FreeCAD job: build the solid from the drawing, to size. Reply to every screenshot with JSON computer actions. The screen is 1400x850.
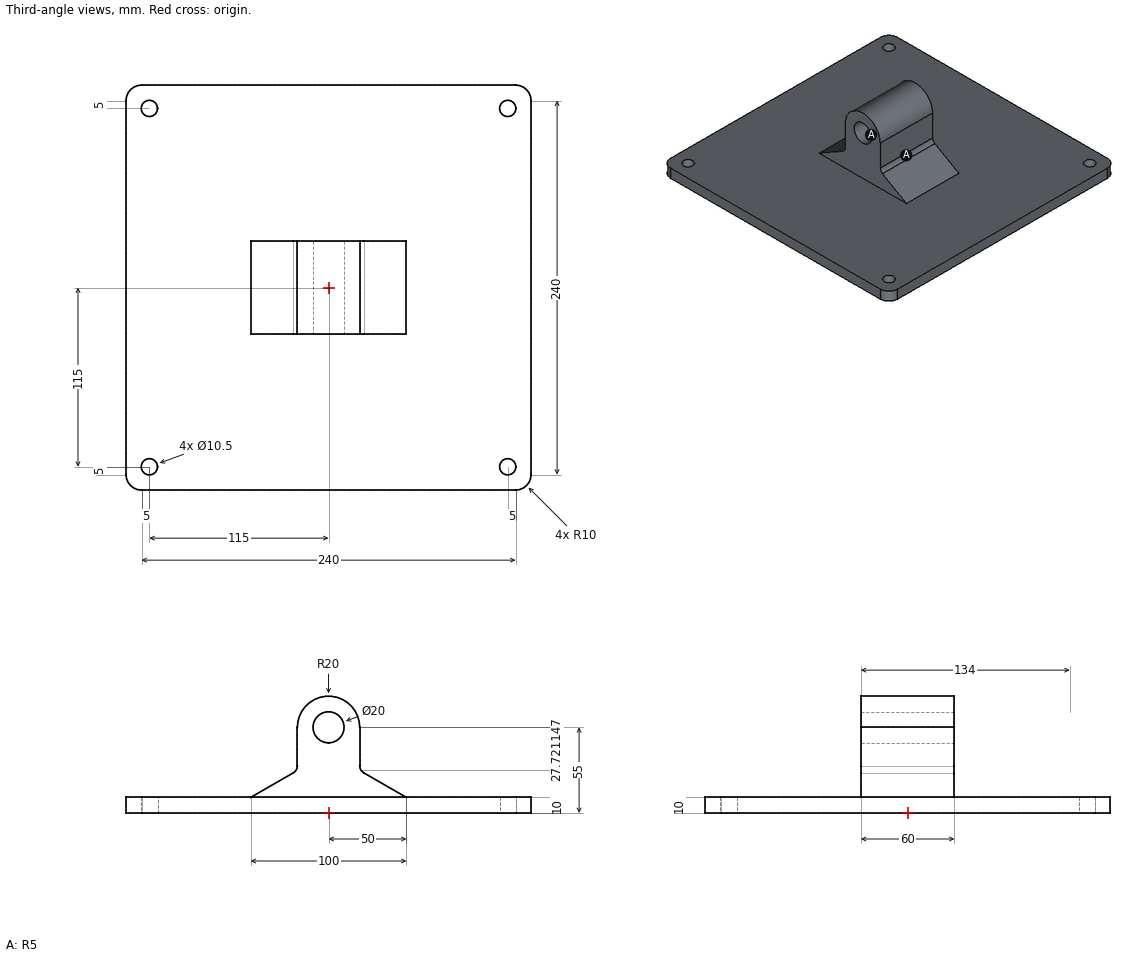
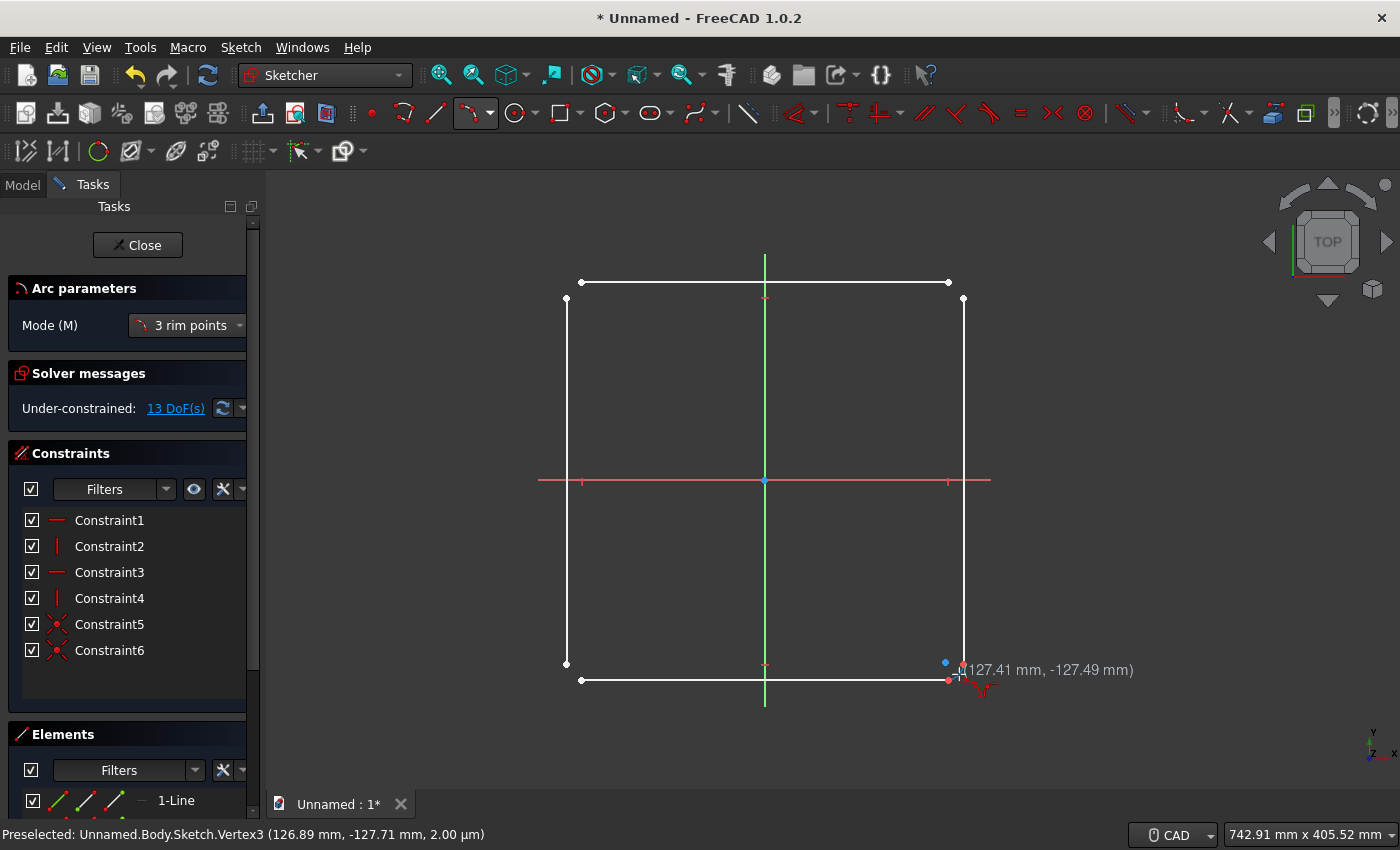
{"action": "left_click", "coordinate": [964, 298]}
{"action": "left_click", "coordinate": [949, 282]}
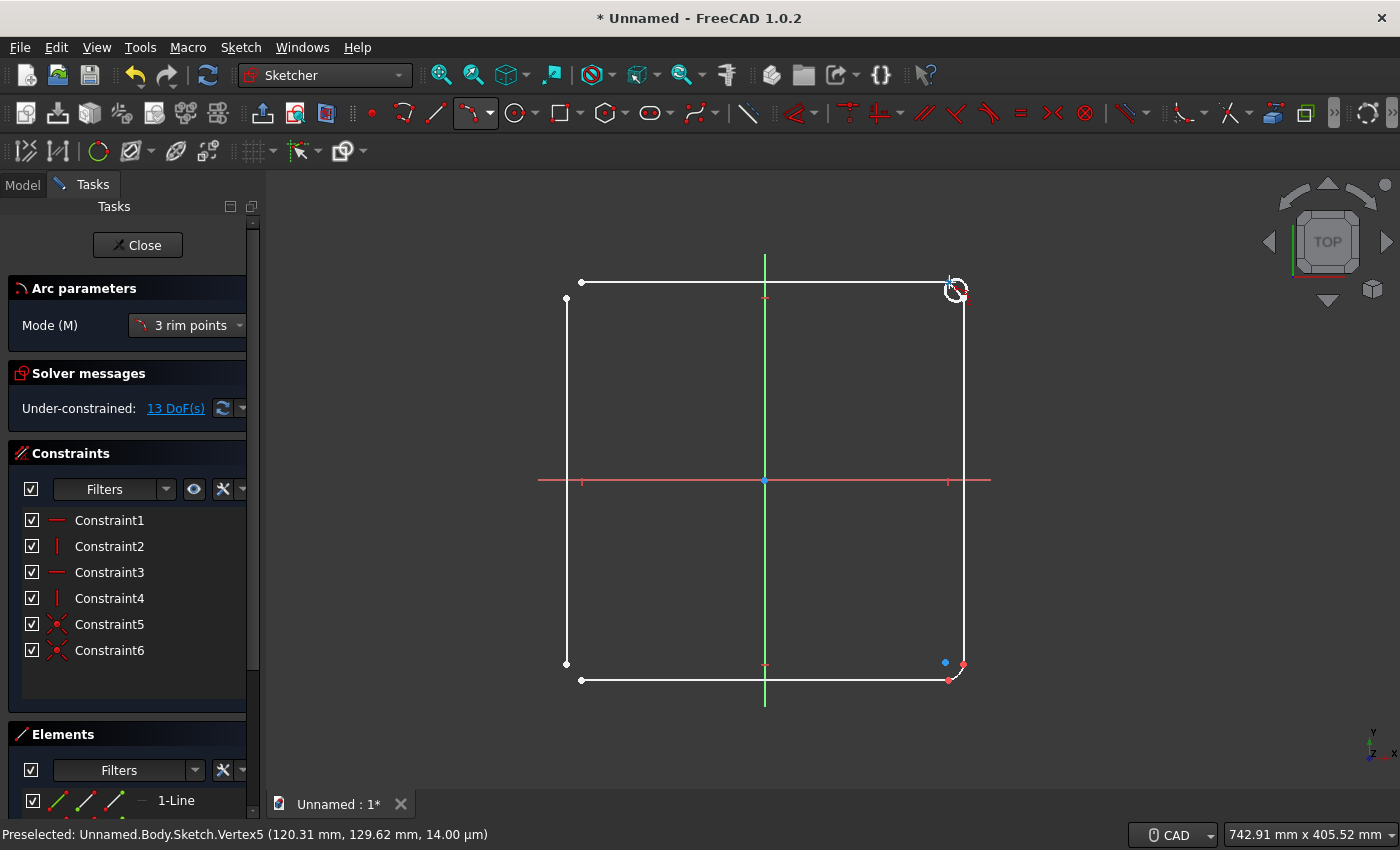
{"action": "scroll", "coordinate": [959, 286], "scroll_direction": "up", "scroll_amount": 7}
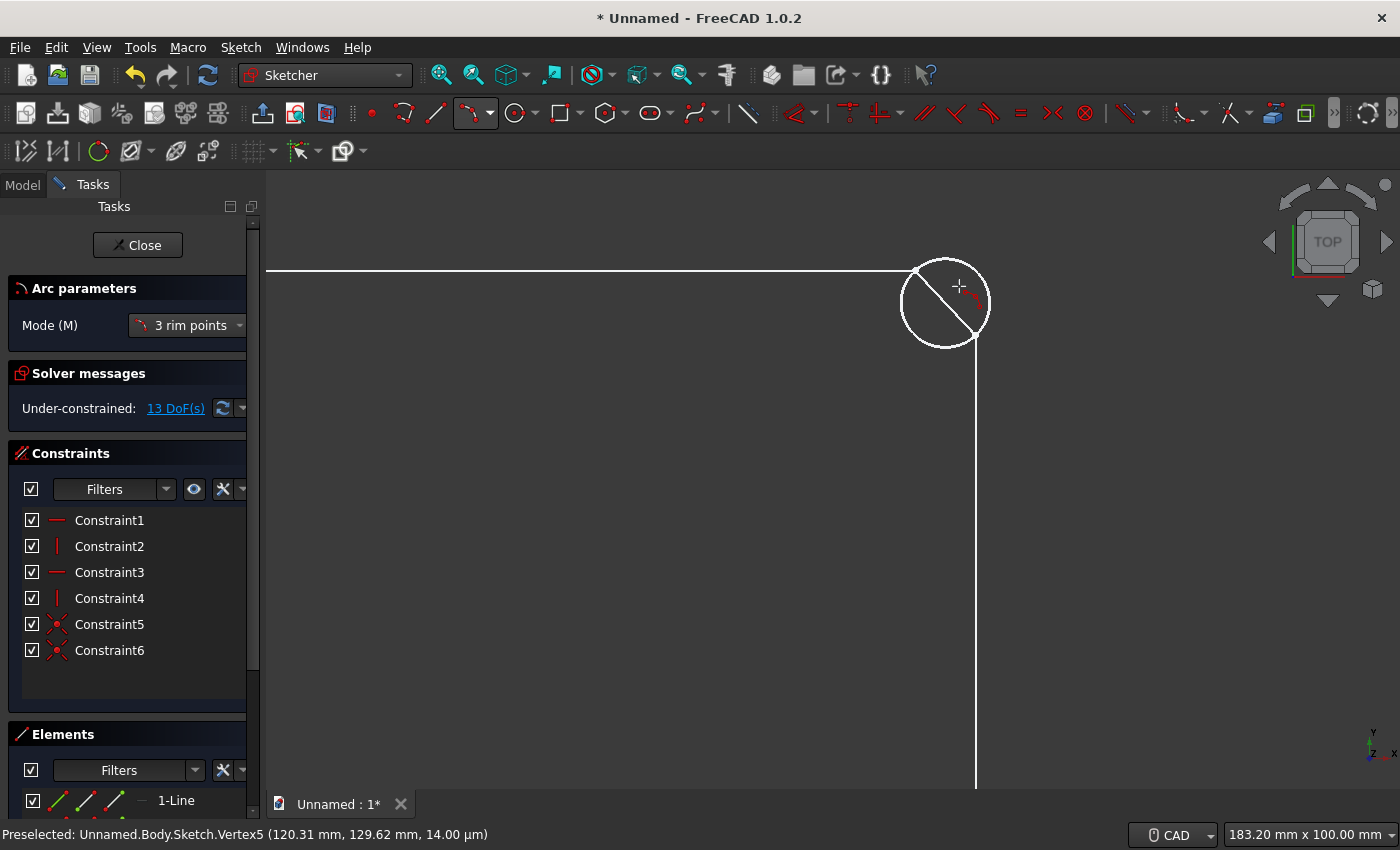
{"action": "left_click", "coordinate": [957, 287]}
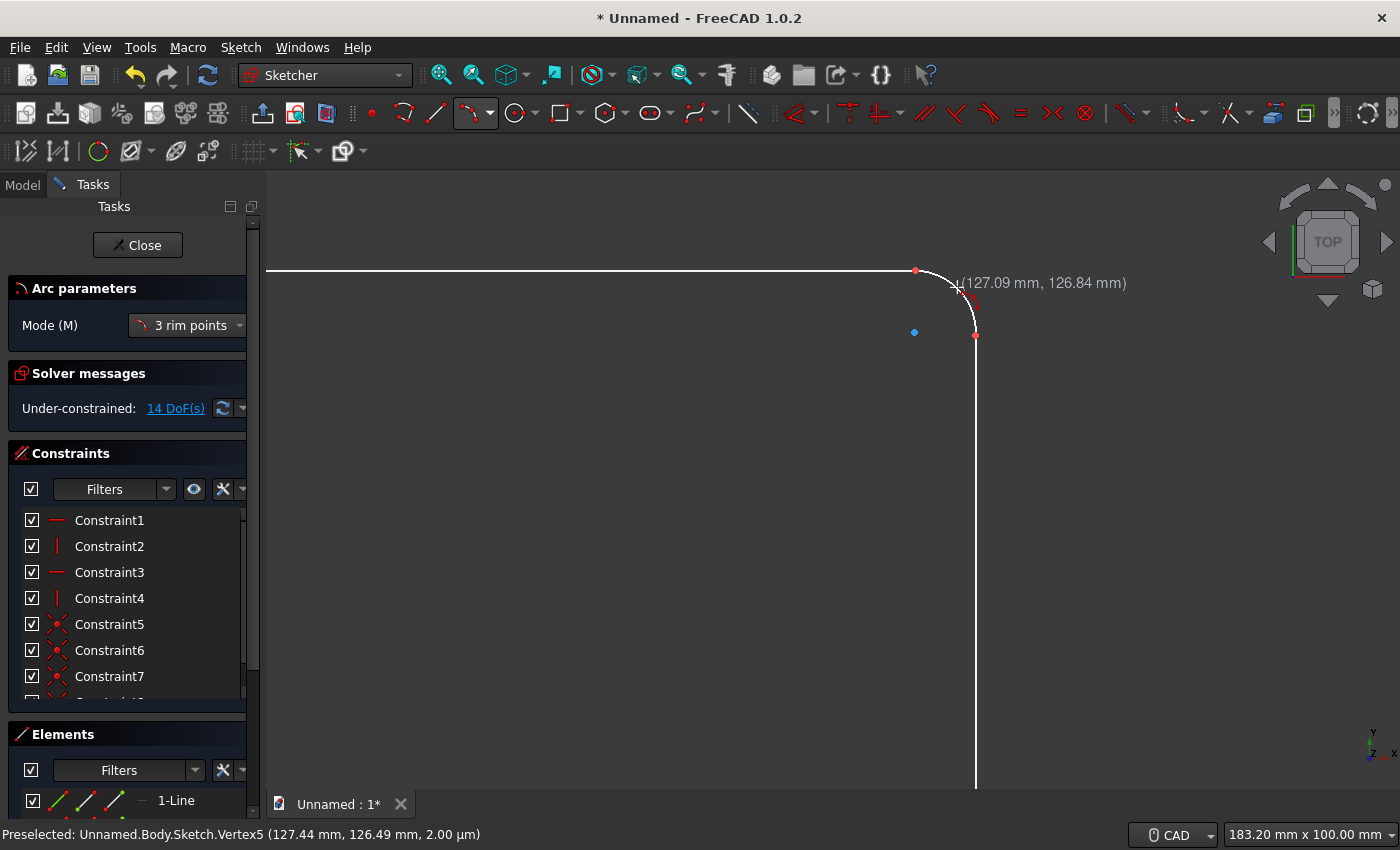
{"action": "scroll", "coordinate": [959, 285], "scroll_direction": "down", "scroll_amount": 7}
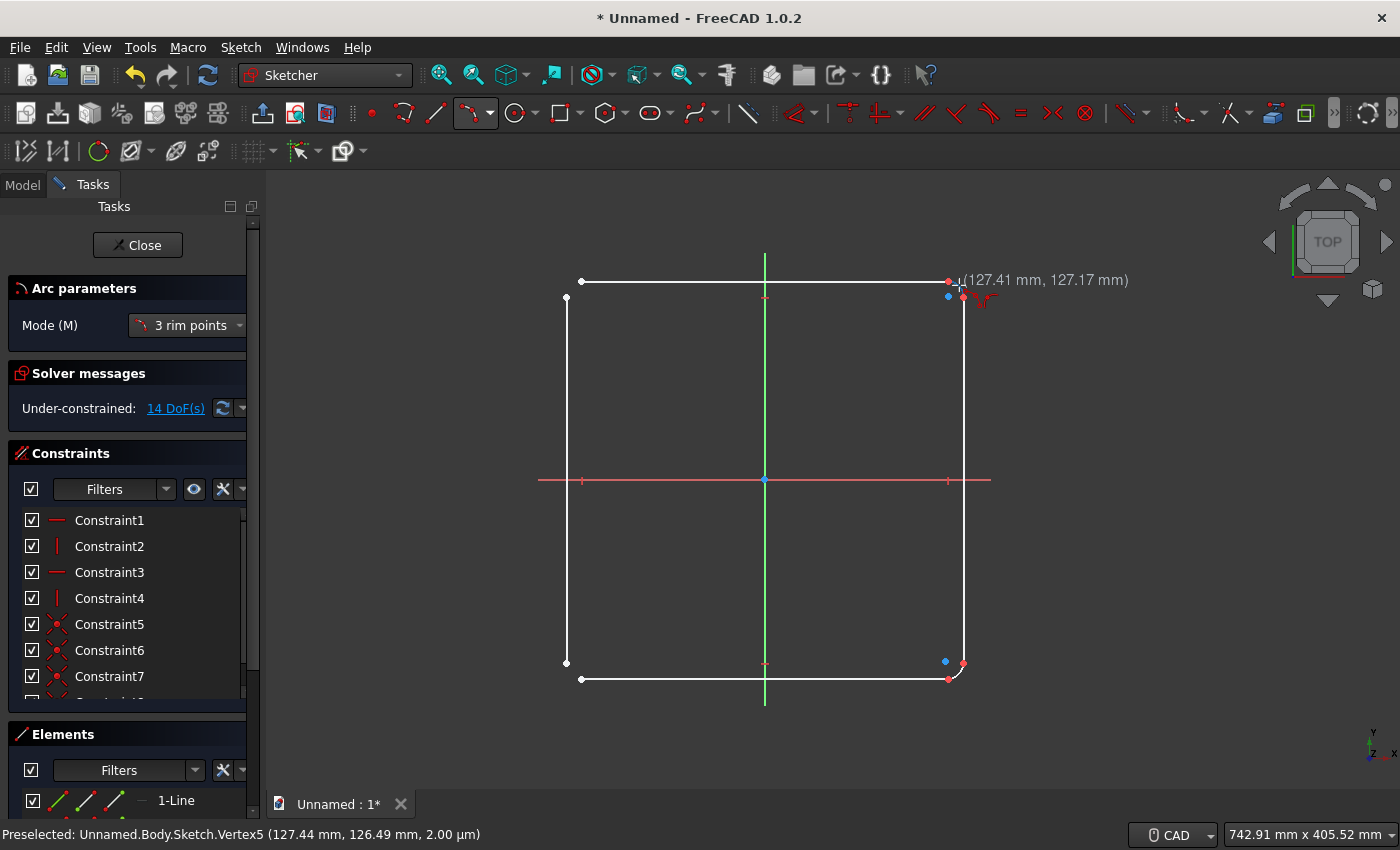
{"action": "left_click", "coordinate": [582, 282]}
{"action": "left_click", "coordinate": [567, 298]}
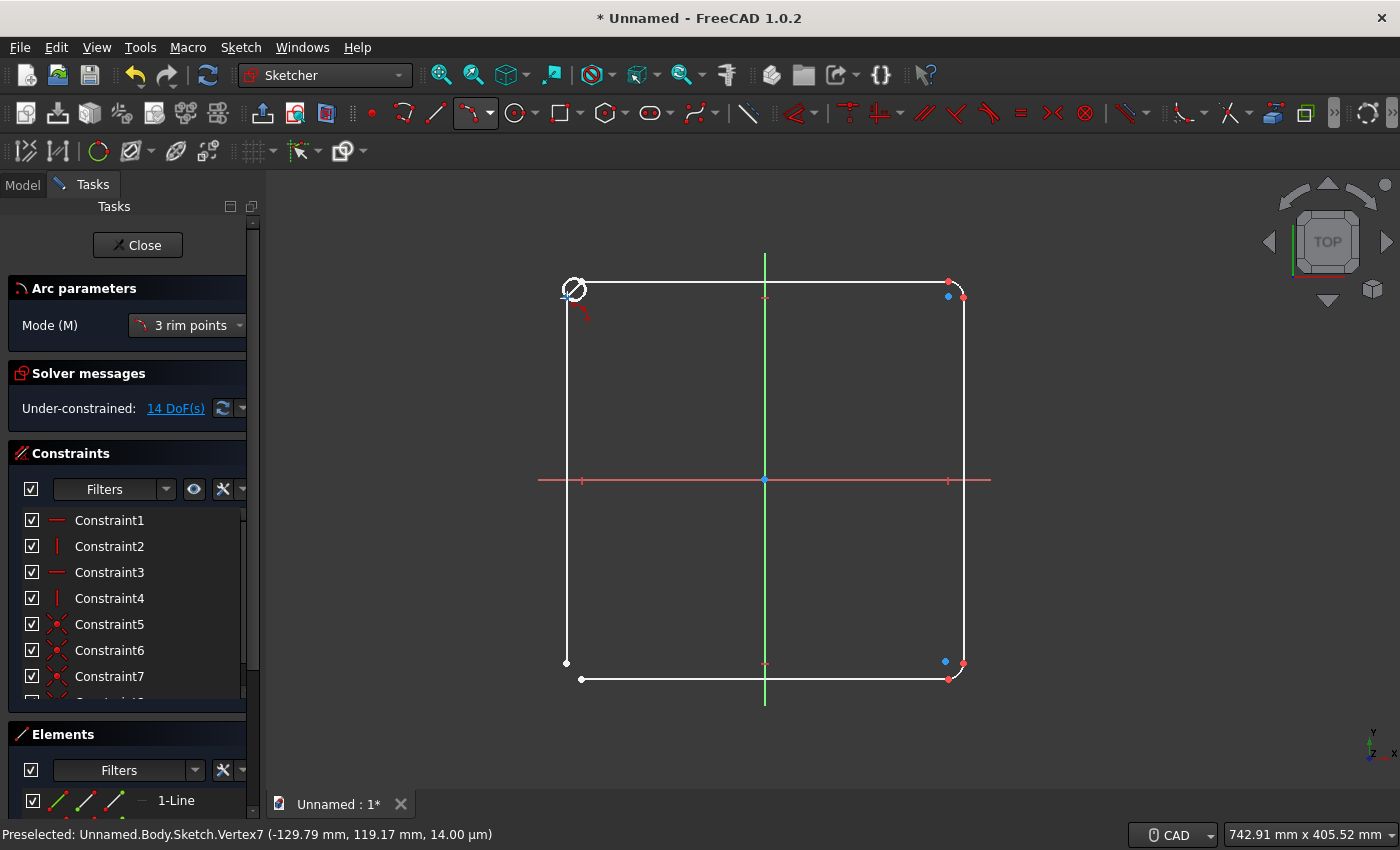
{"action": "scroll", "coordinate": [571, 286], "scroll_direction": "up", "scroll_amount": 7}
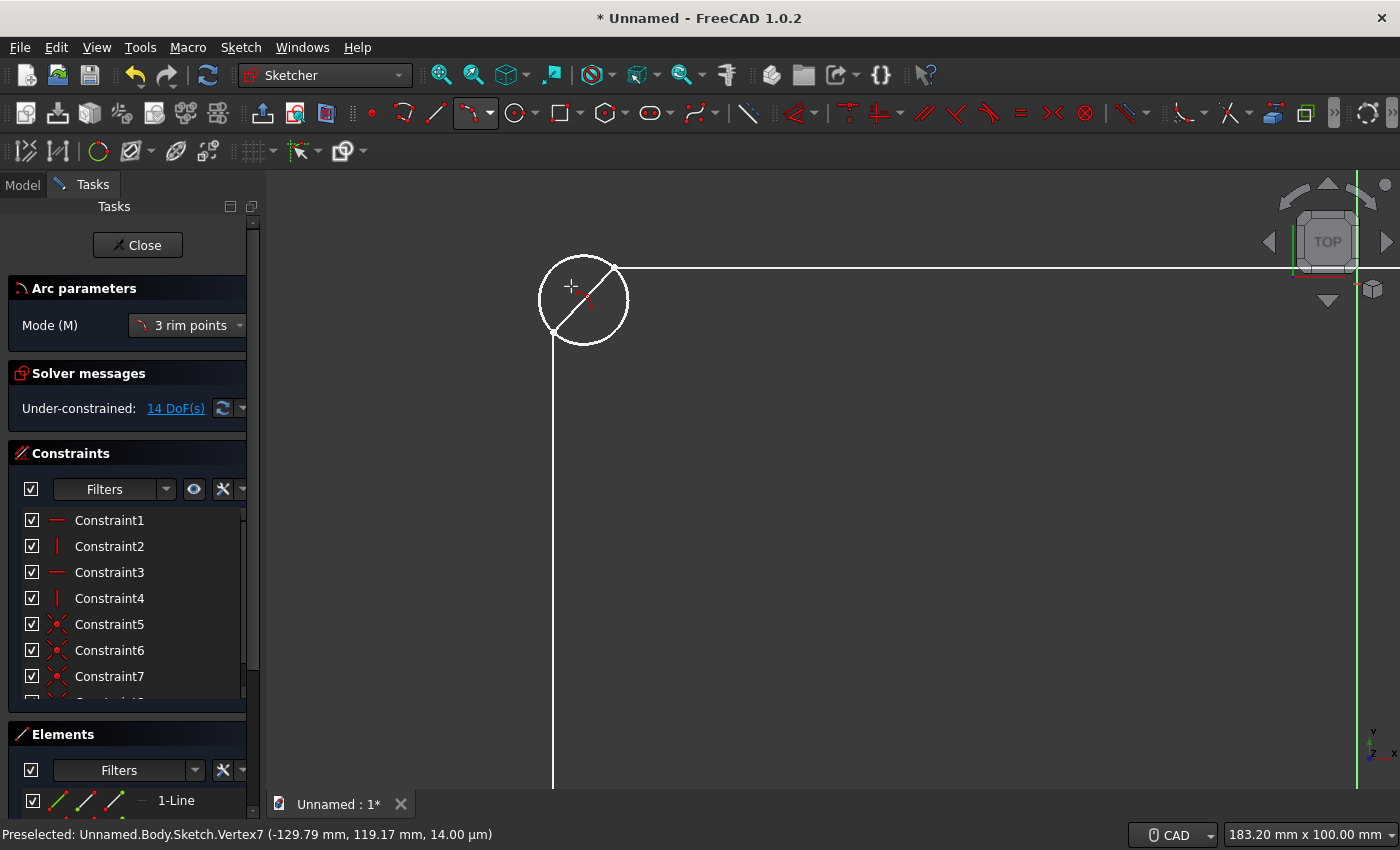
{"action": "left_click", "coordinate": [570, 284]}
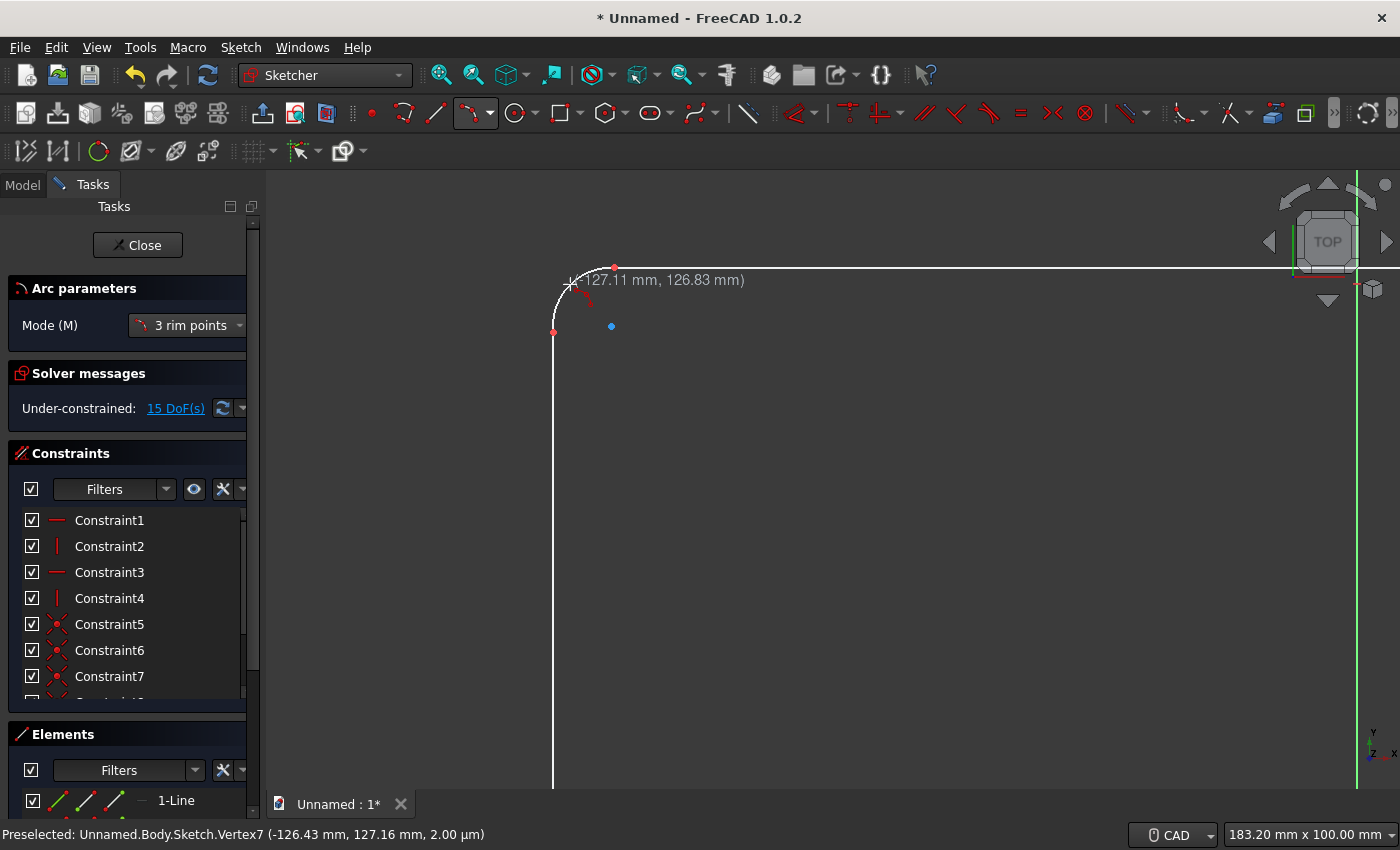
{"action": "scroll", "coordinate": [571, 286], "scroll_direction": "down", "scroll_amount": 7}